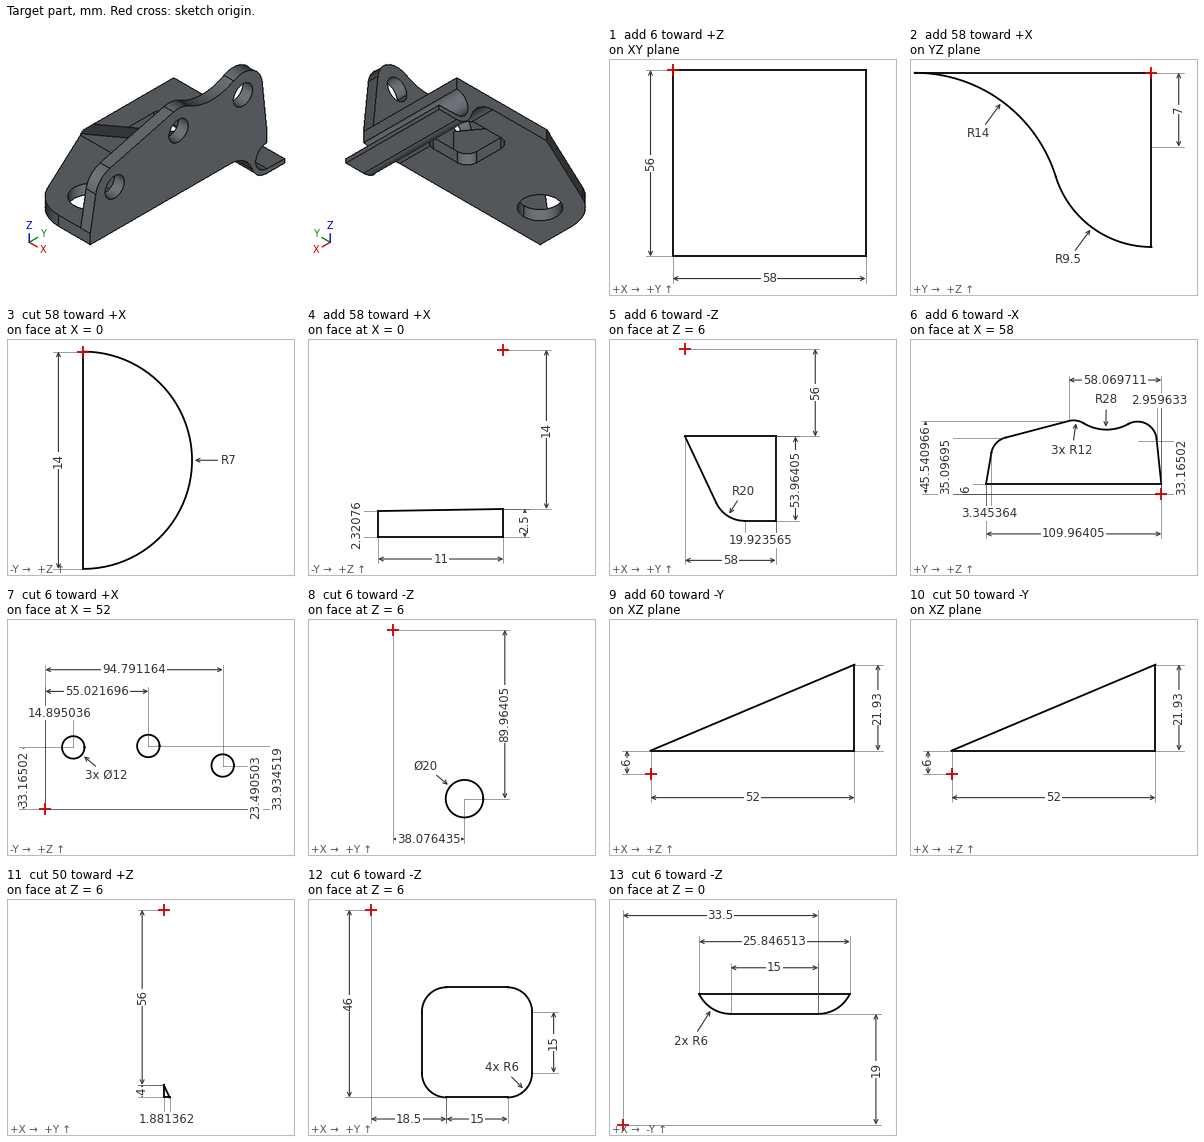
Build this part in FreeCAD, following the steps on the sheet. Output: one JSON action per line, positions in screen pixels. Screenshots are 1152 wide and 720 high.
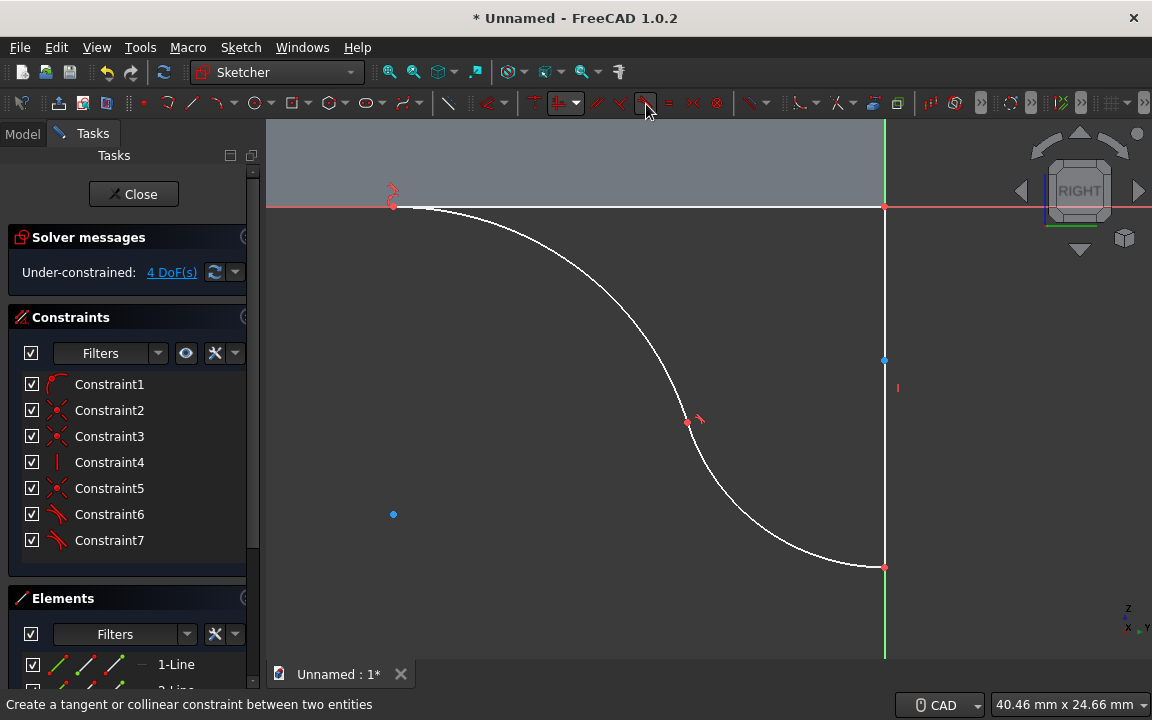
{"action": "left_click", "coordinate": [885, 361]}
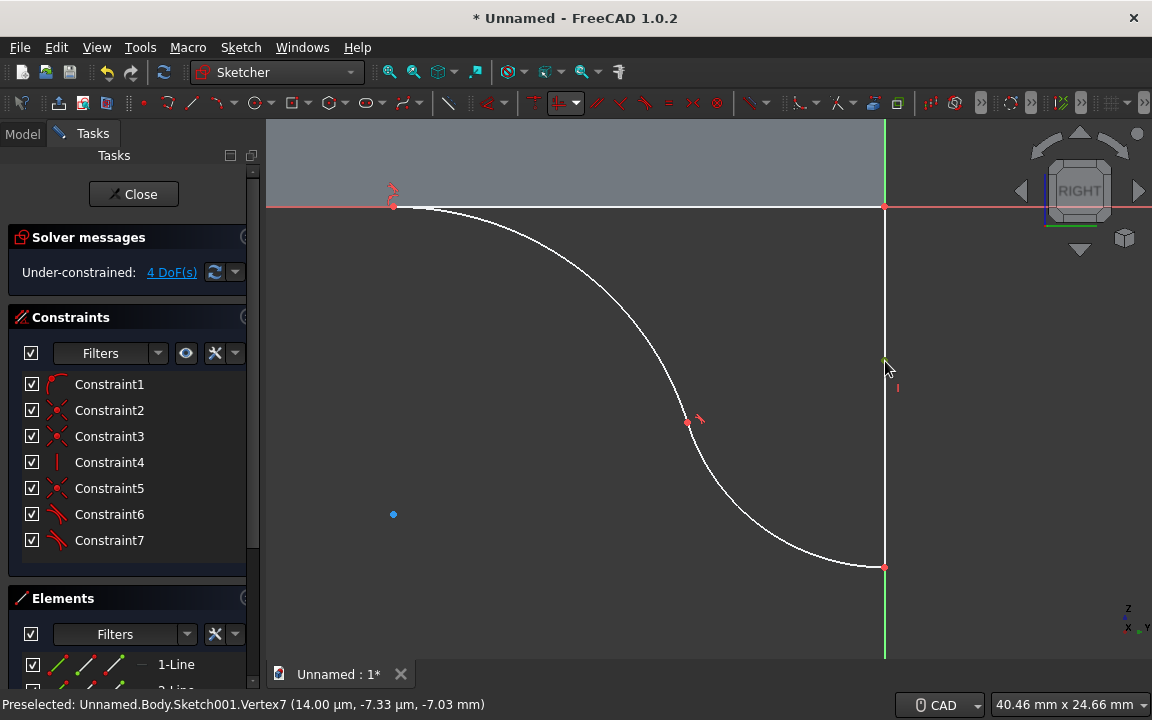
{"action": "left_click", "coordinate": [885, 596]}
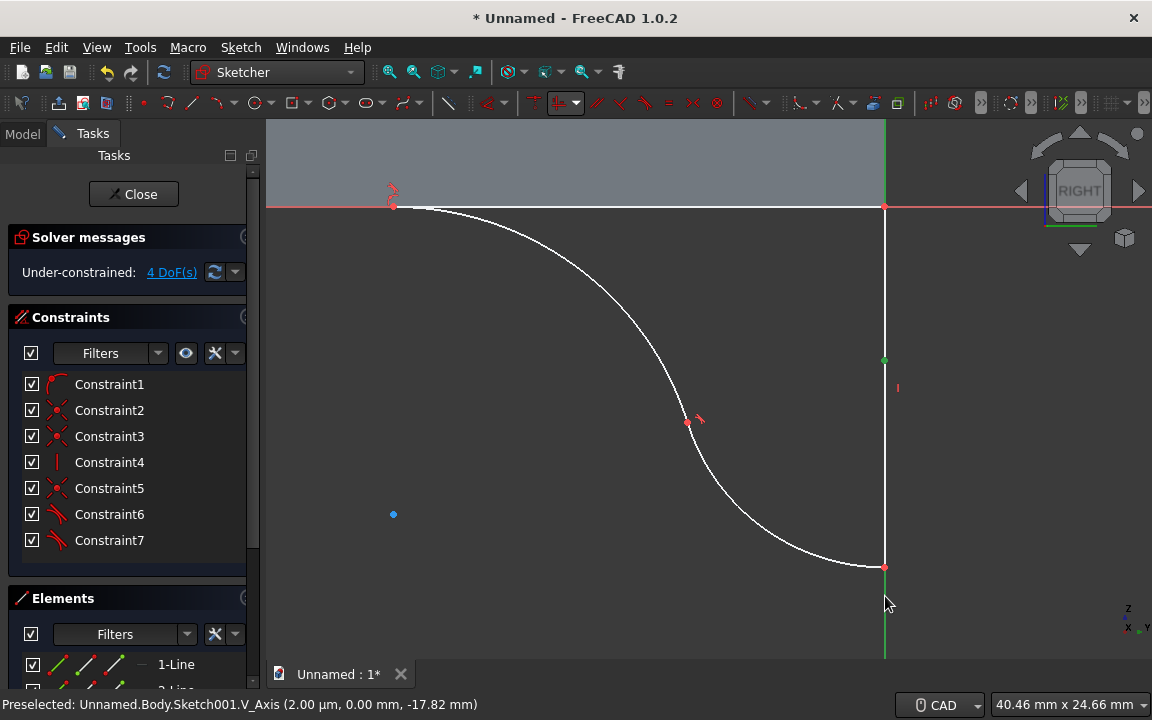
{"action": "key", "text": "c"}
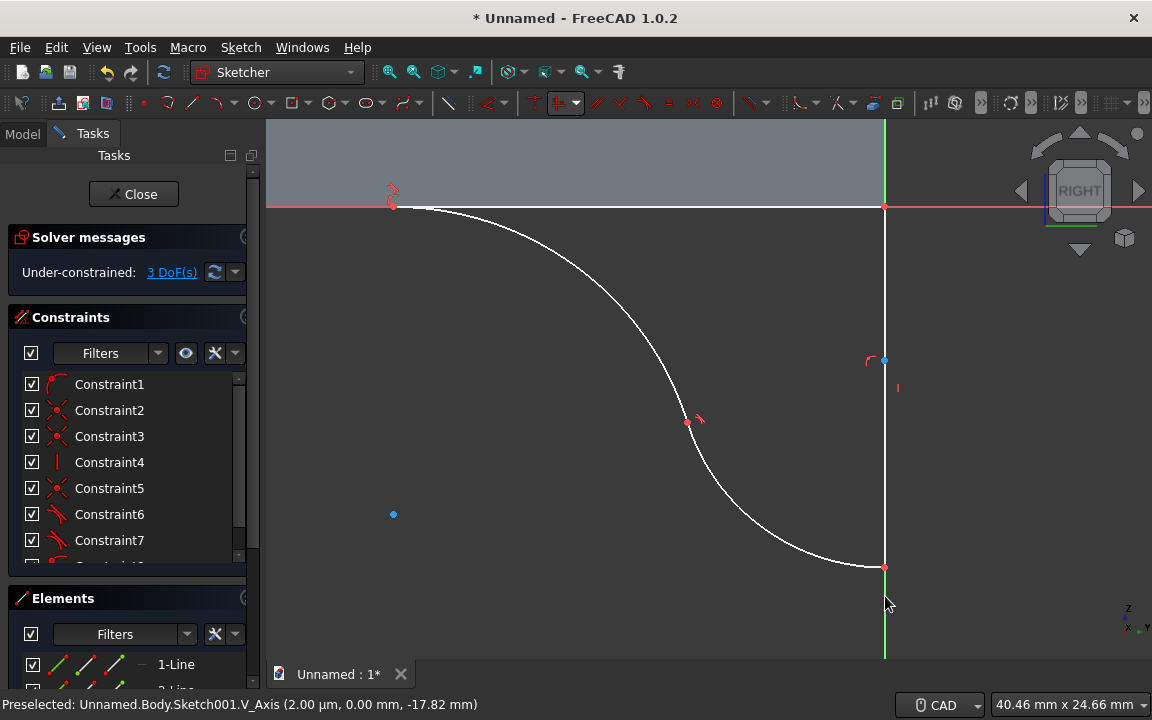
{"action": "left_click", "coordinate": [488, 104]}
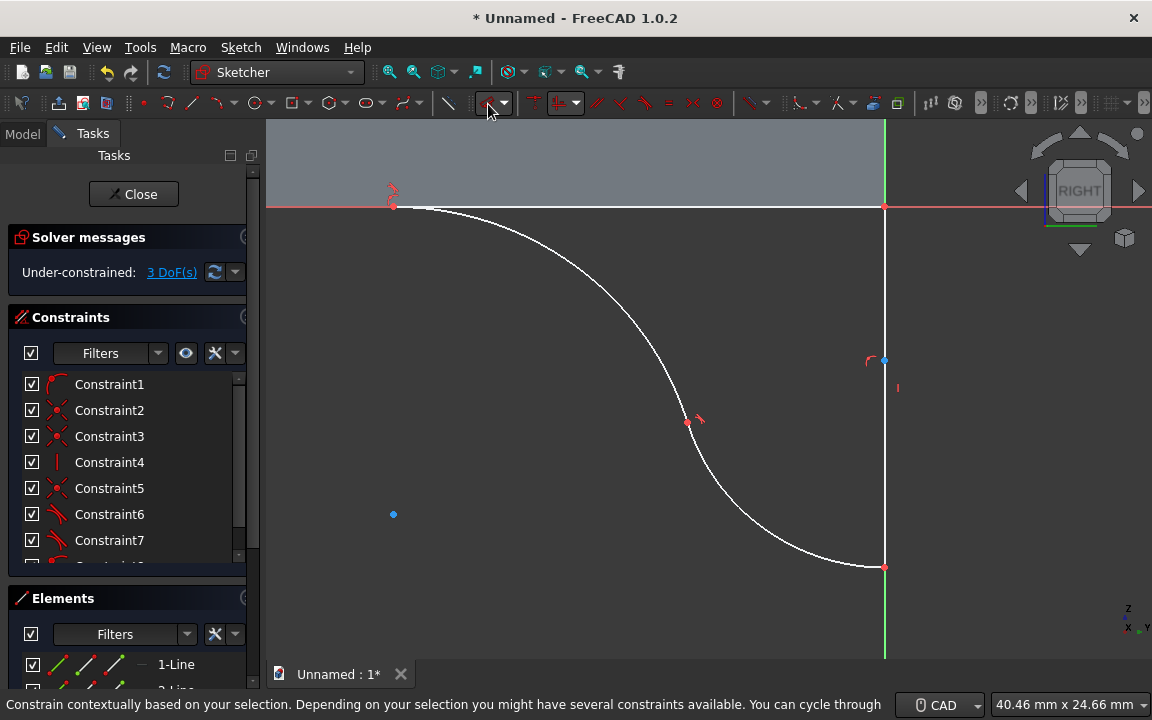
{"action": "left_click", "coordinate": [725, 491]}
{"action": "left_click", "coordinate": [700, 511]}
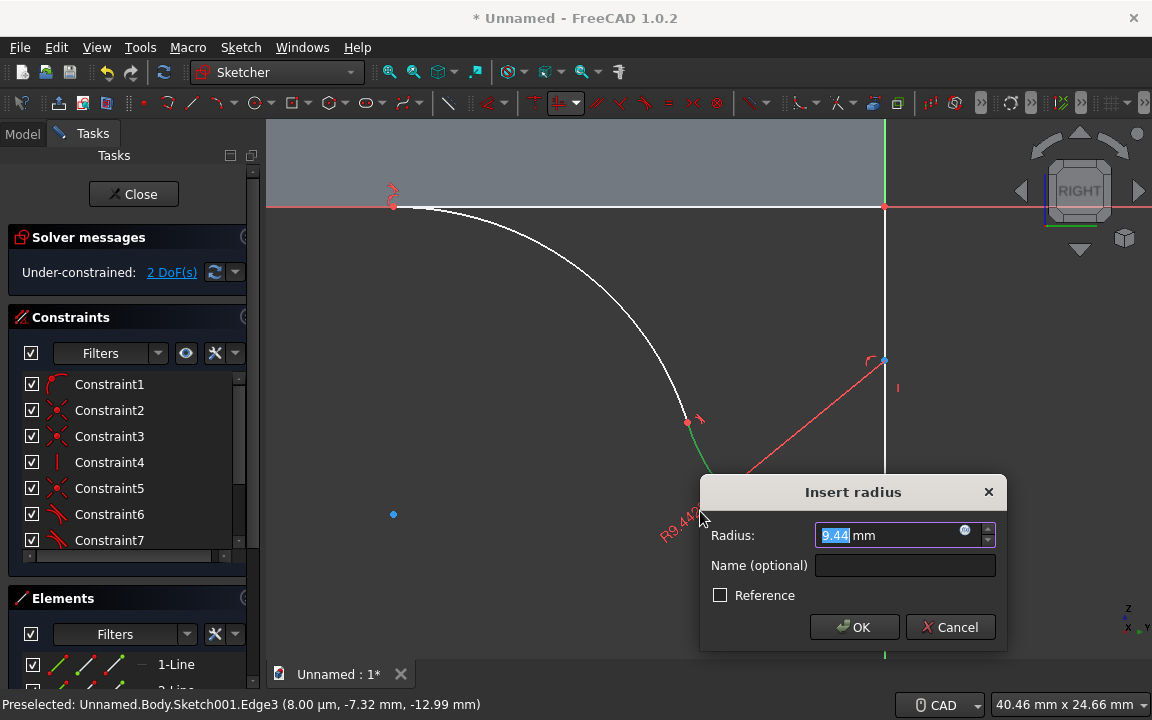
{"action": "type", "text": "9.5"}
{"action": "key", "text": "Return"}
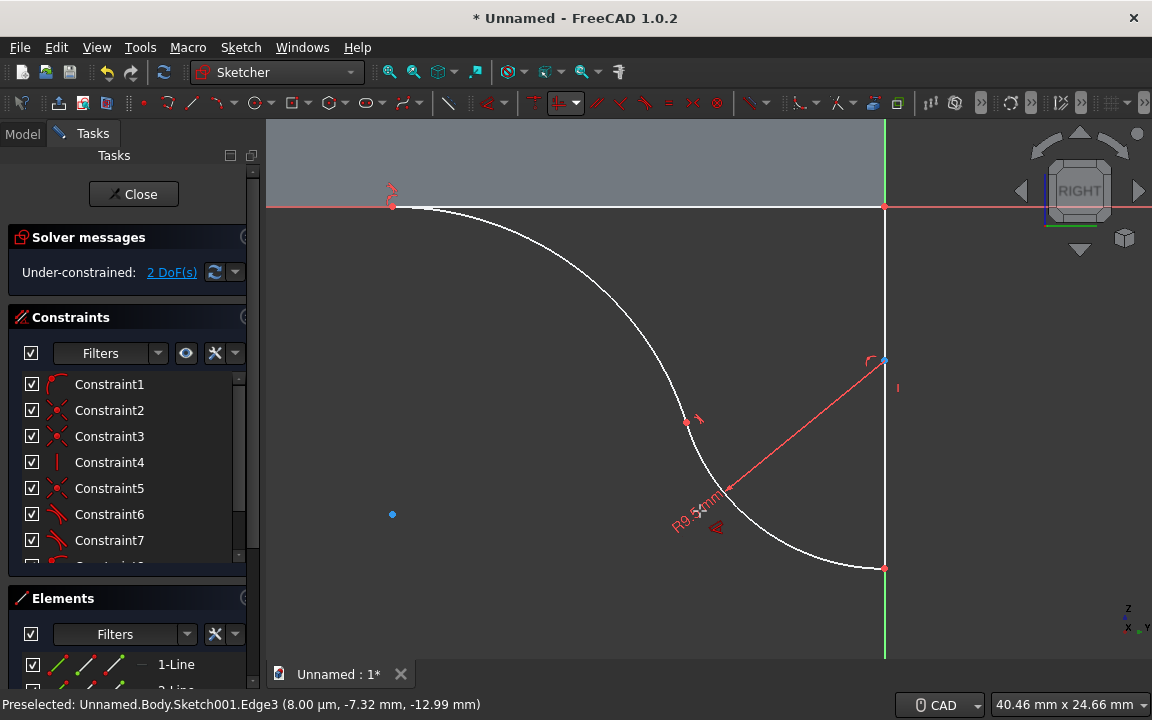
{"action": "left_click", "coordinate": [631, 320]}
{"action": "left_click", "coordinate": [656, 300]}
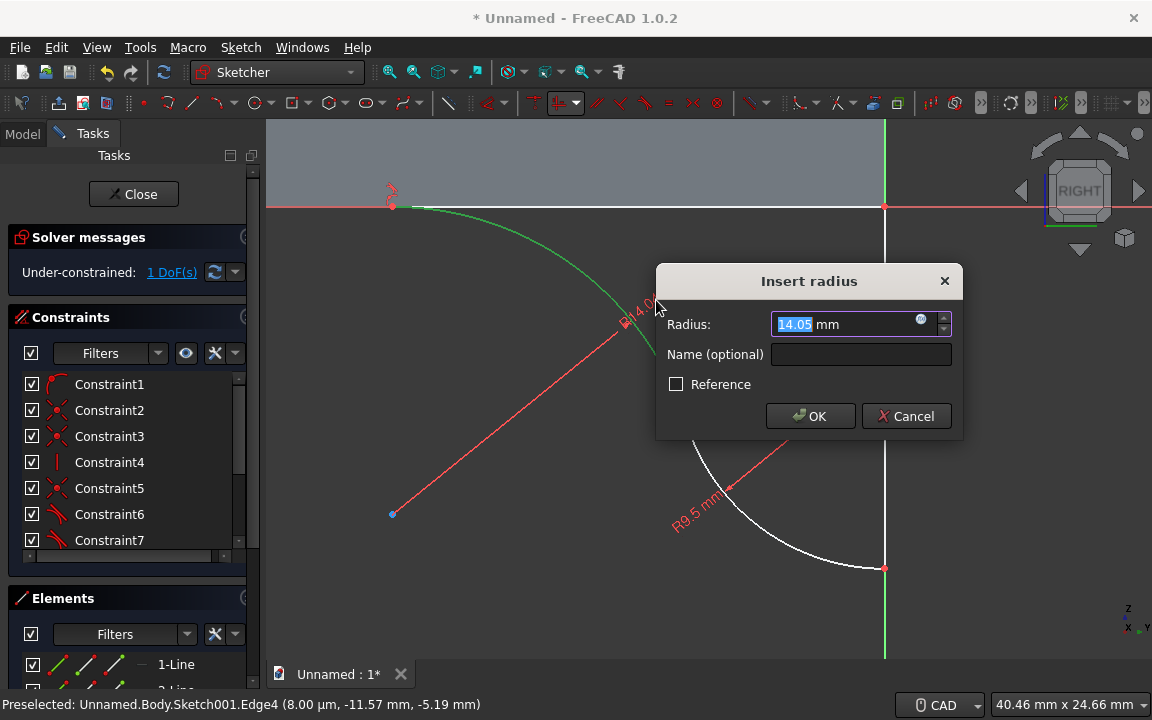
{"action": "type", "text": "14"}
{"action": "key", "text": "Return"}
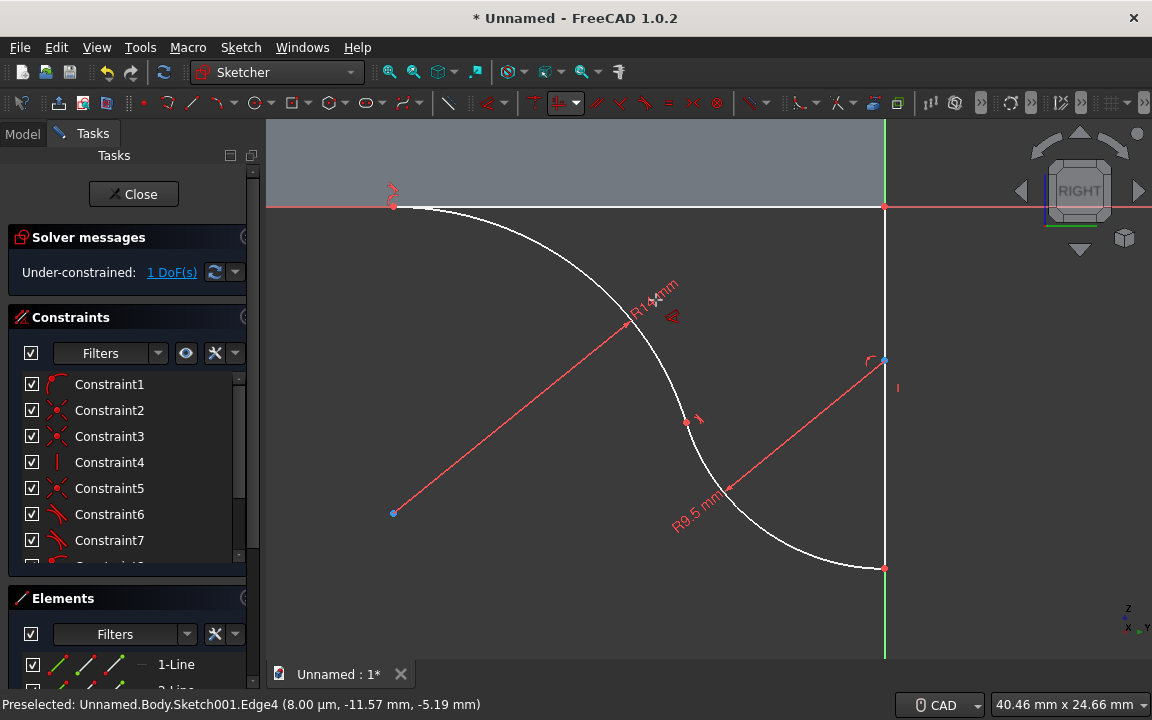
{"action": "left_click", "coordinate": [885, 361]}
{"action": "left_click", "coordinate": [919, 284]}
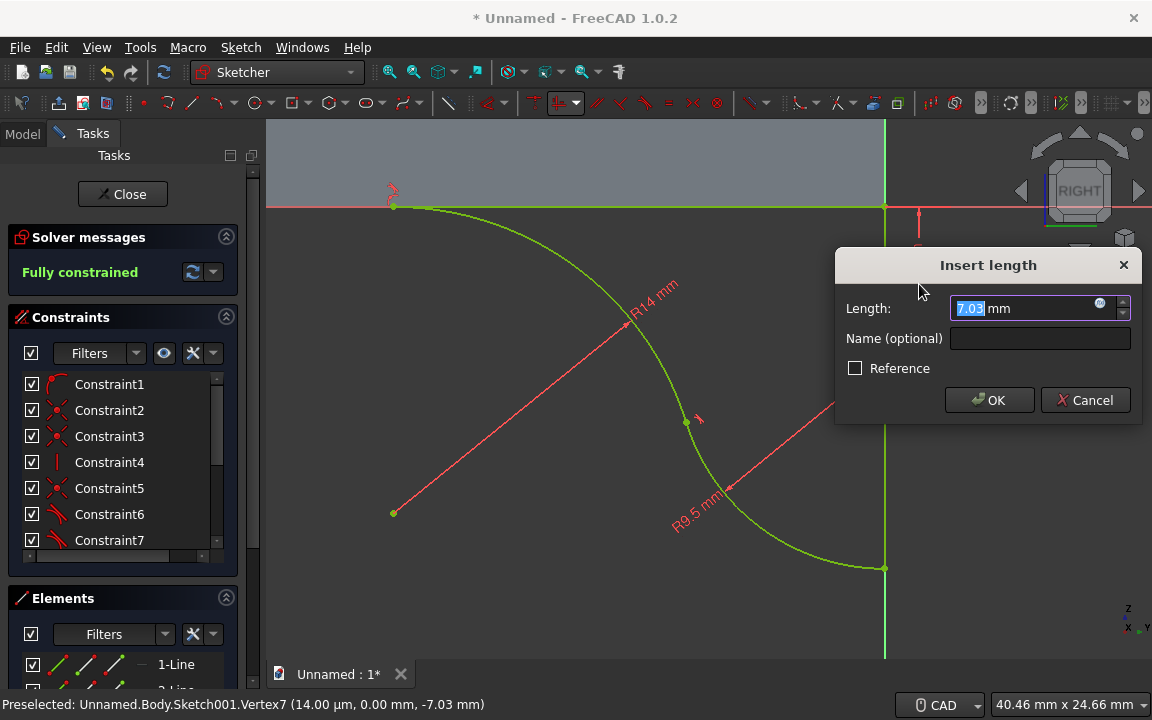
{"action": "type", "text": "7"}
{"action": "key", "text": "Return"}
{"action": "key", "text": "Escape"}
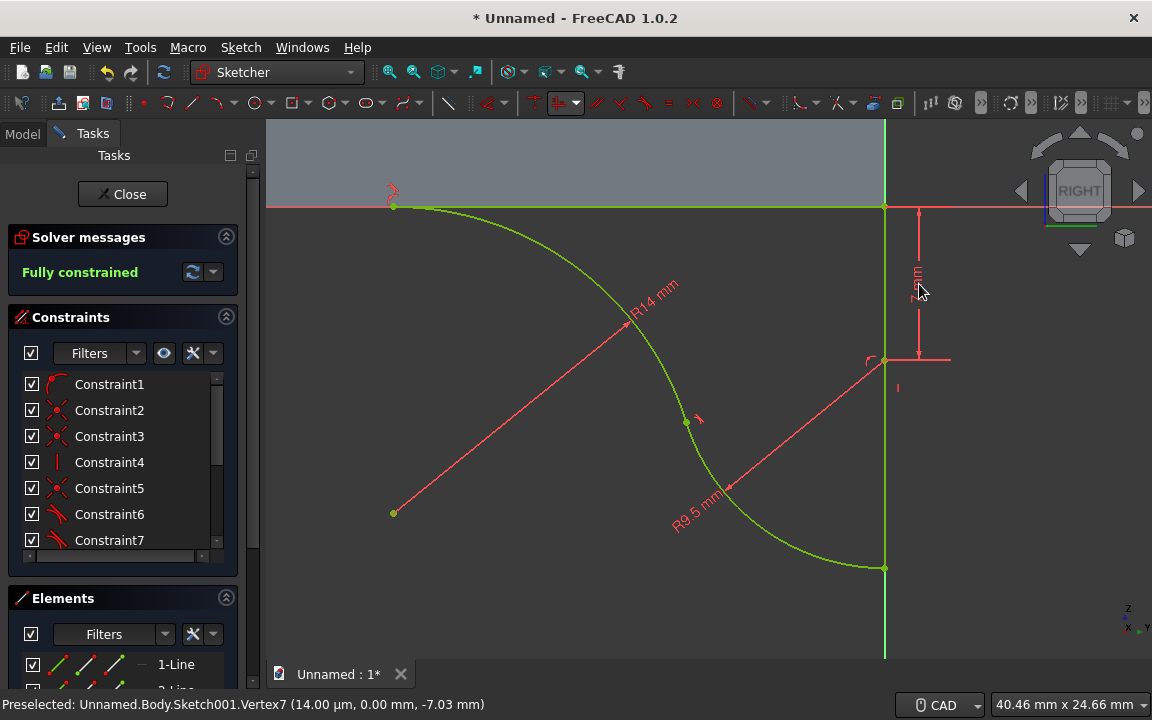
{"action": "left_click", "coordinate": [123, 194]}